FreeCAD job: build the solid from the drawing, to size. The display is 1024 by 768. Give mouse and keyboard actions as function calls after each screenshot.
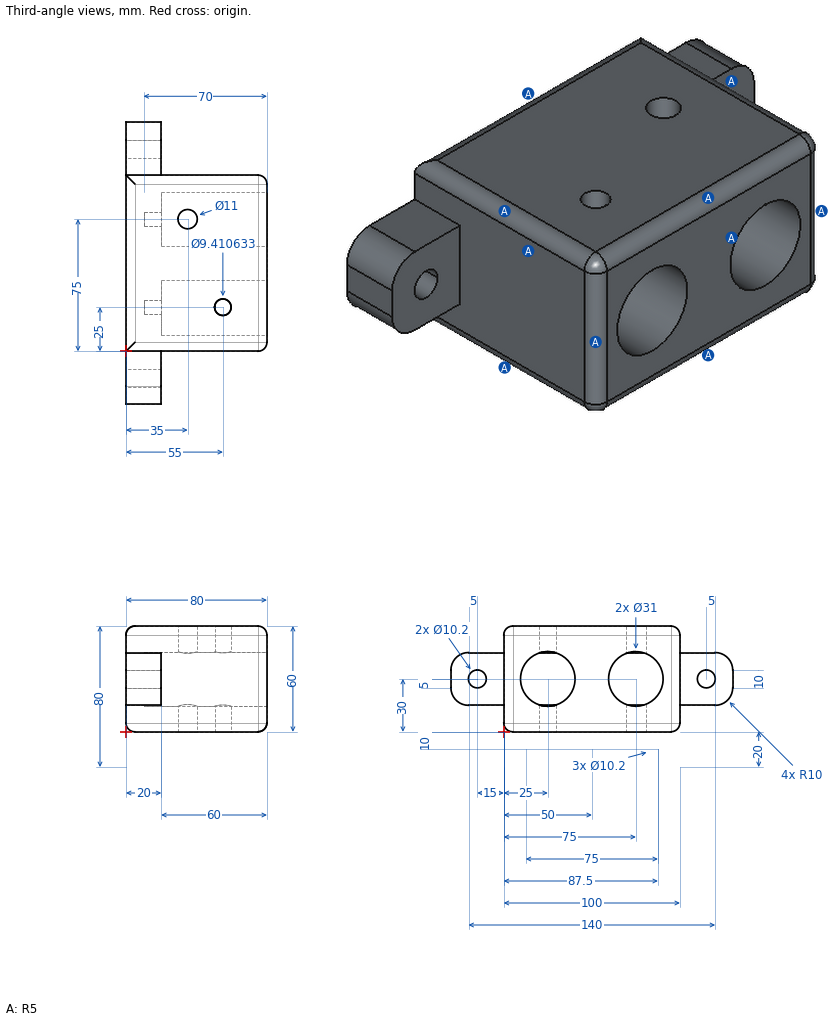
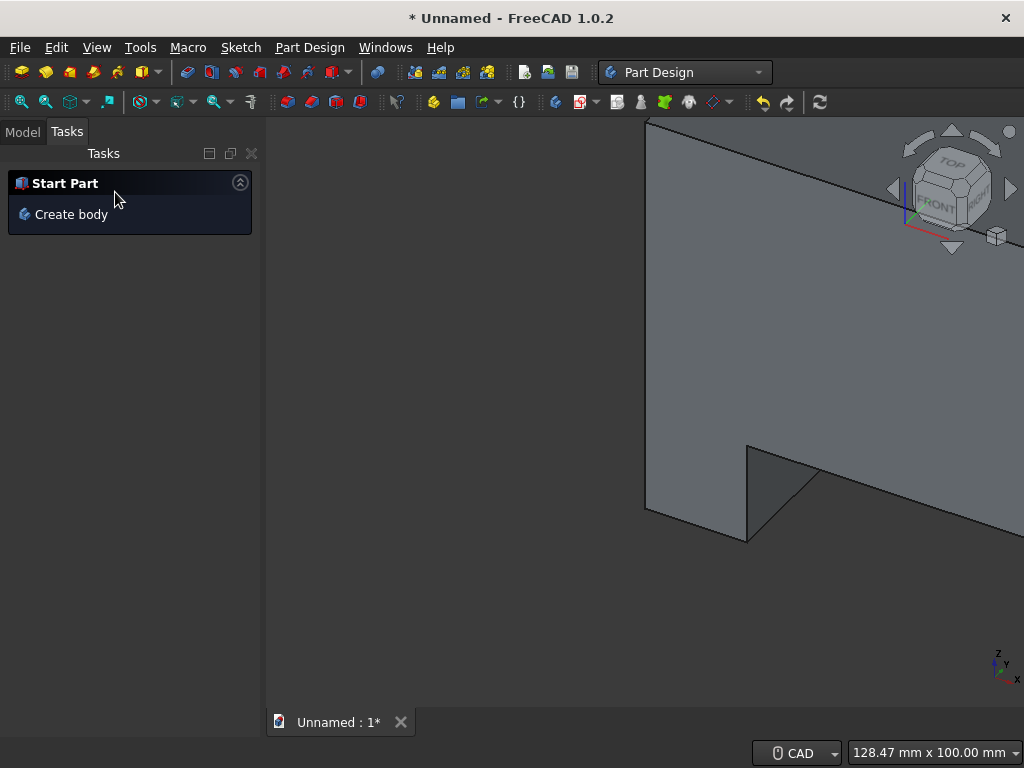
key(v)
key(f)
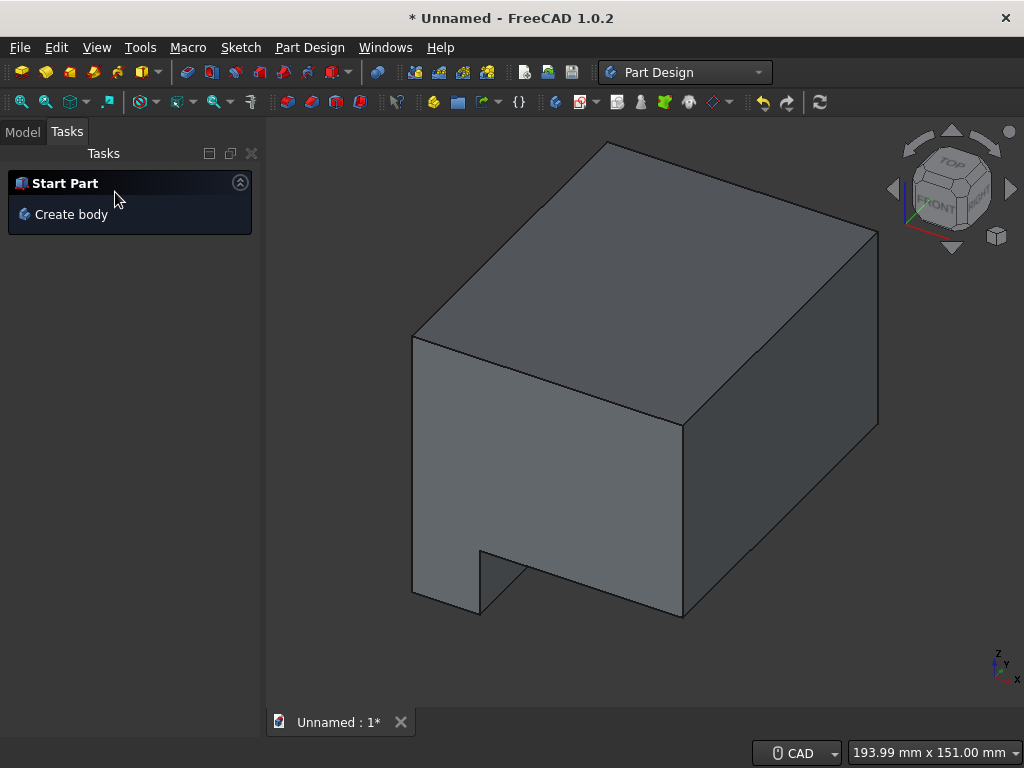
click(808, 396)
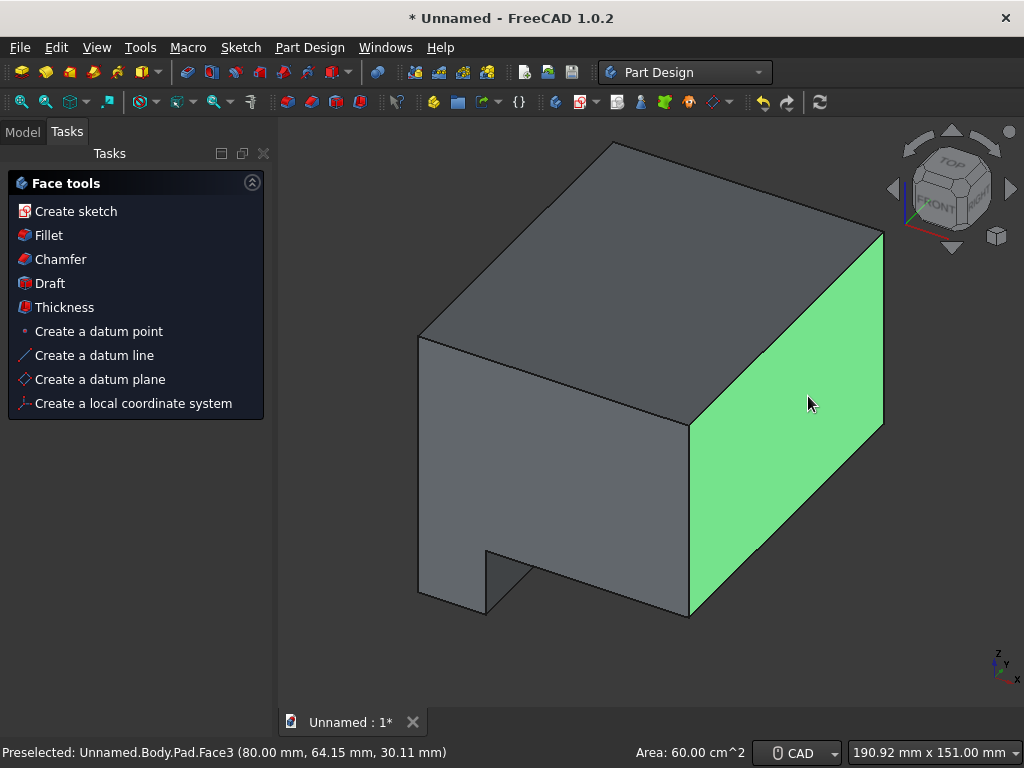
click(580, 102)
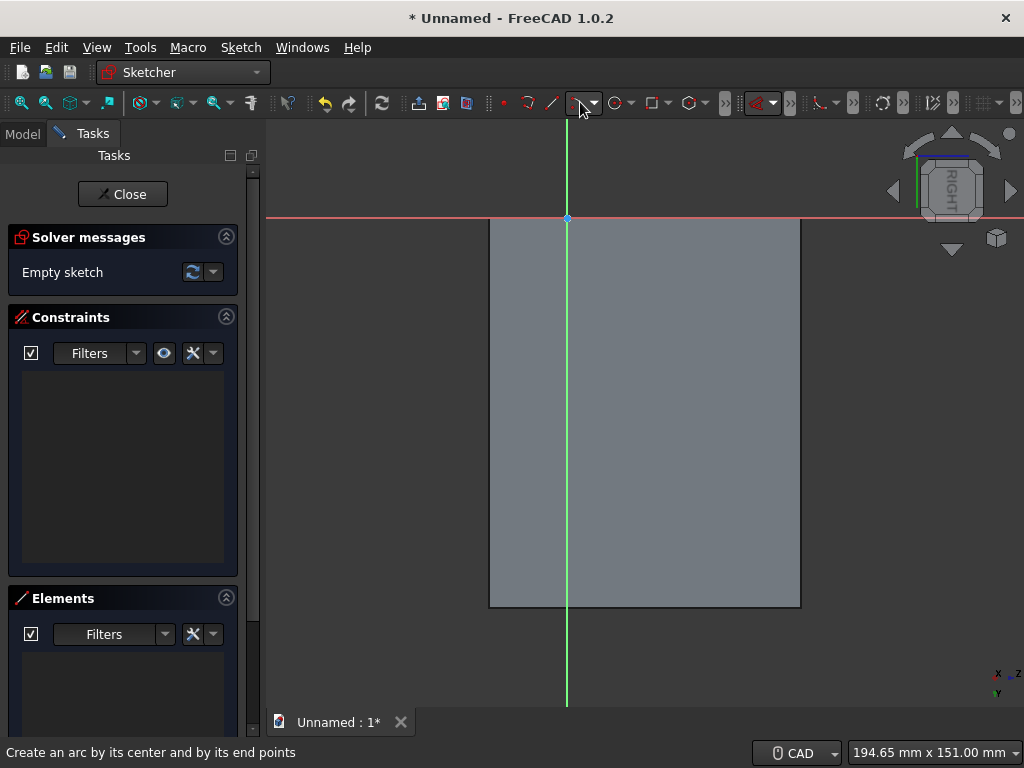
key(g)
key(c)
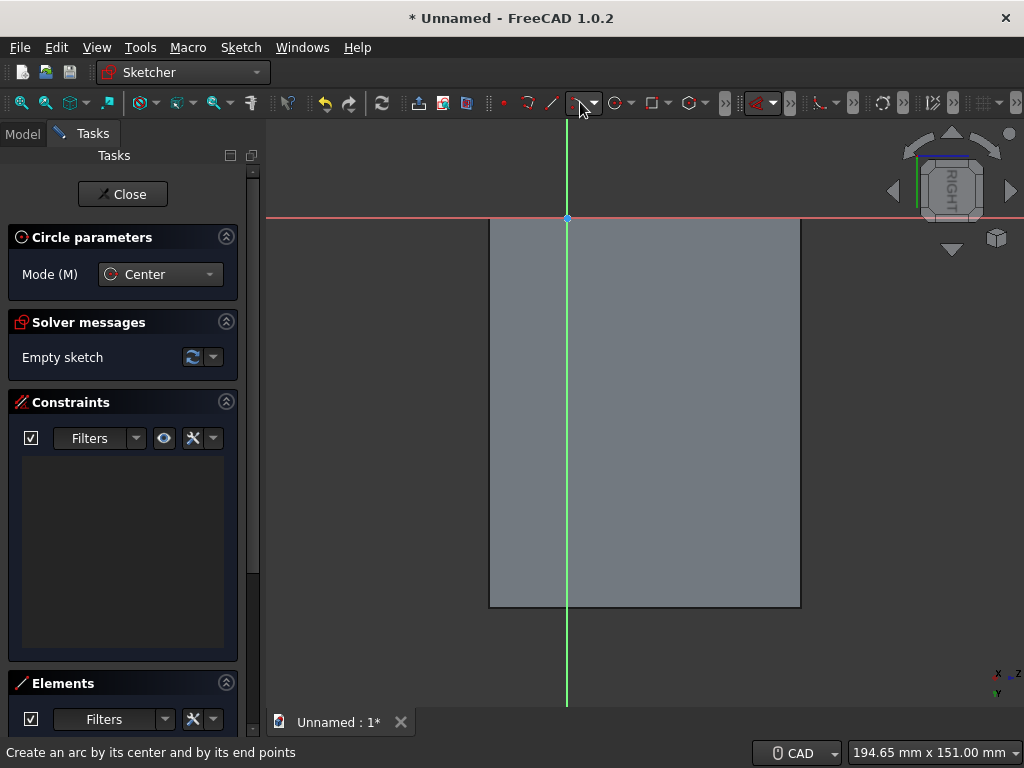
click(684, 510)
move(727, 468)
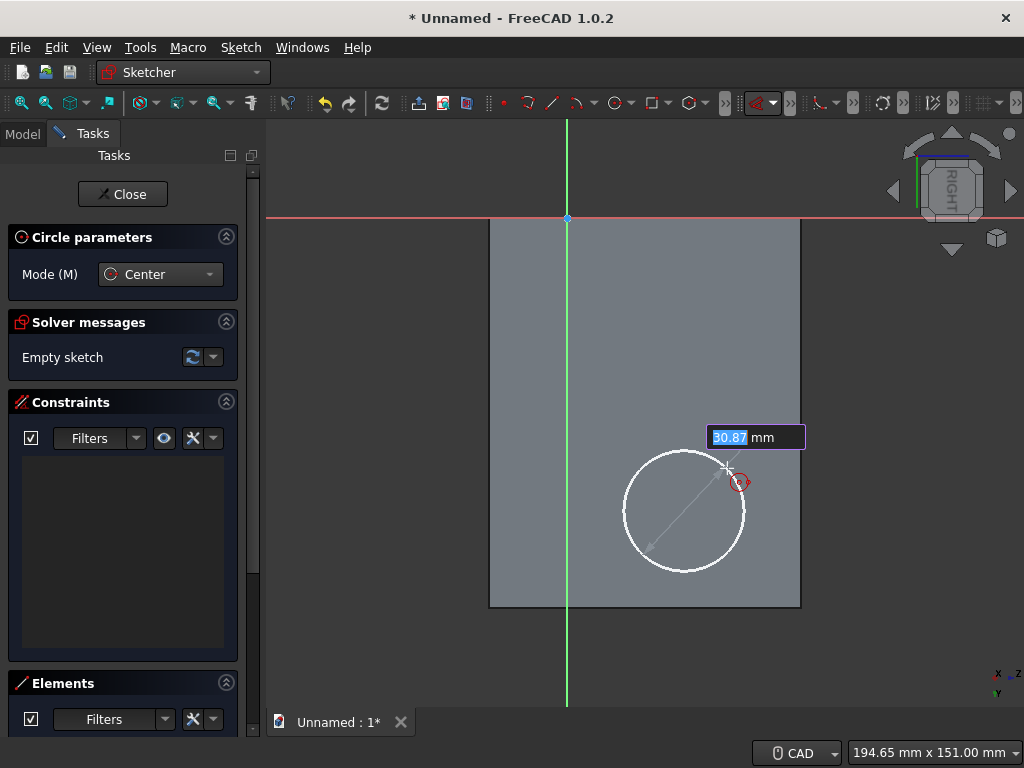
text(31)
key(Return)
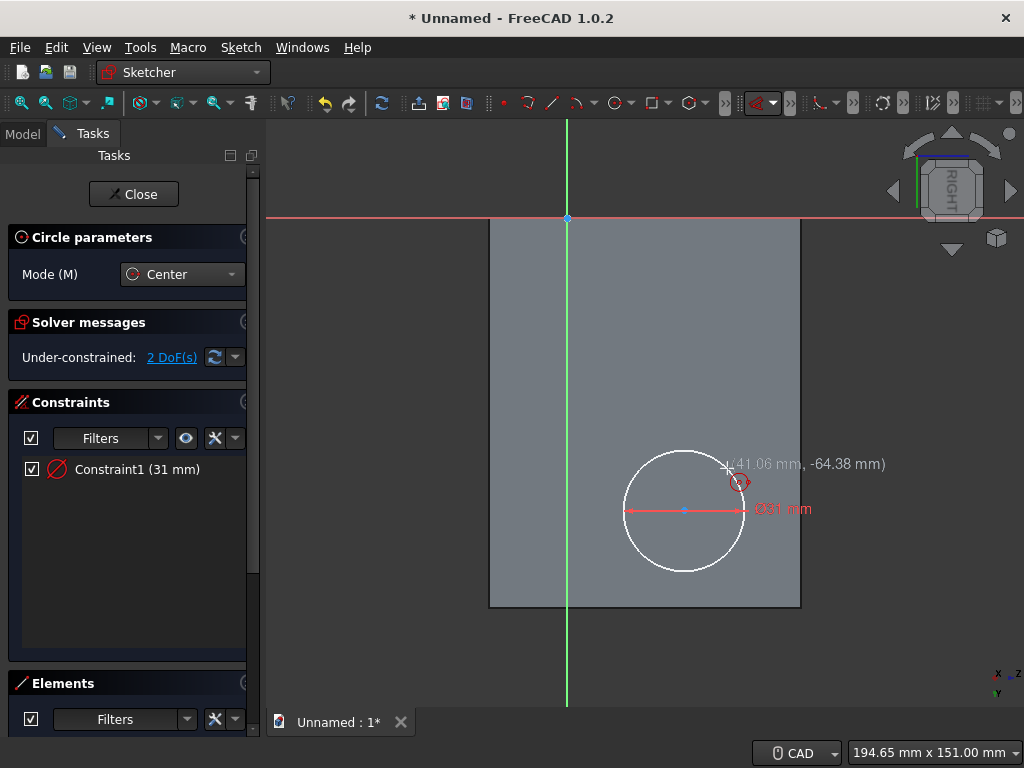
click(684, 316)
move(727, 273)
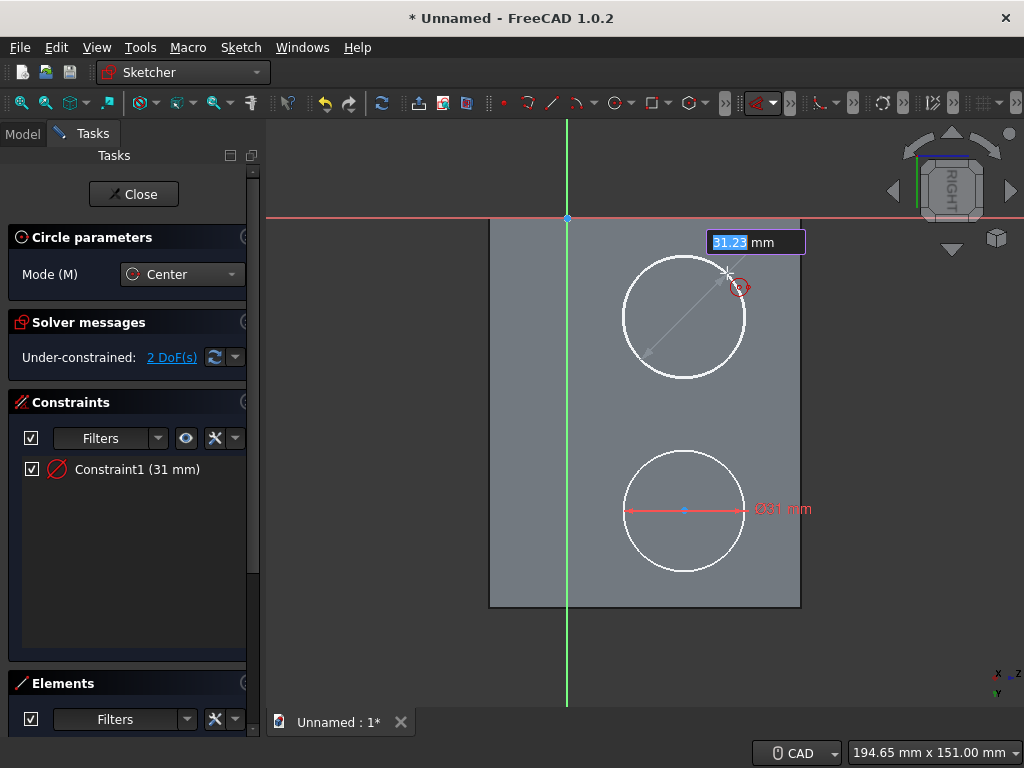
text(31)
key(Return)
key(Escape)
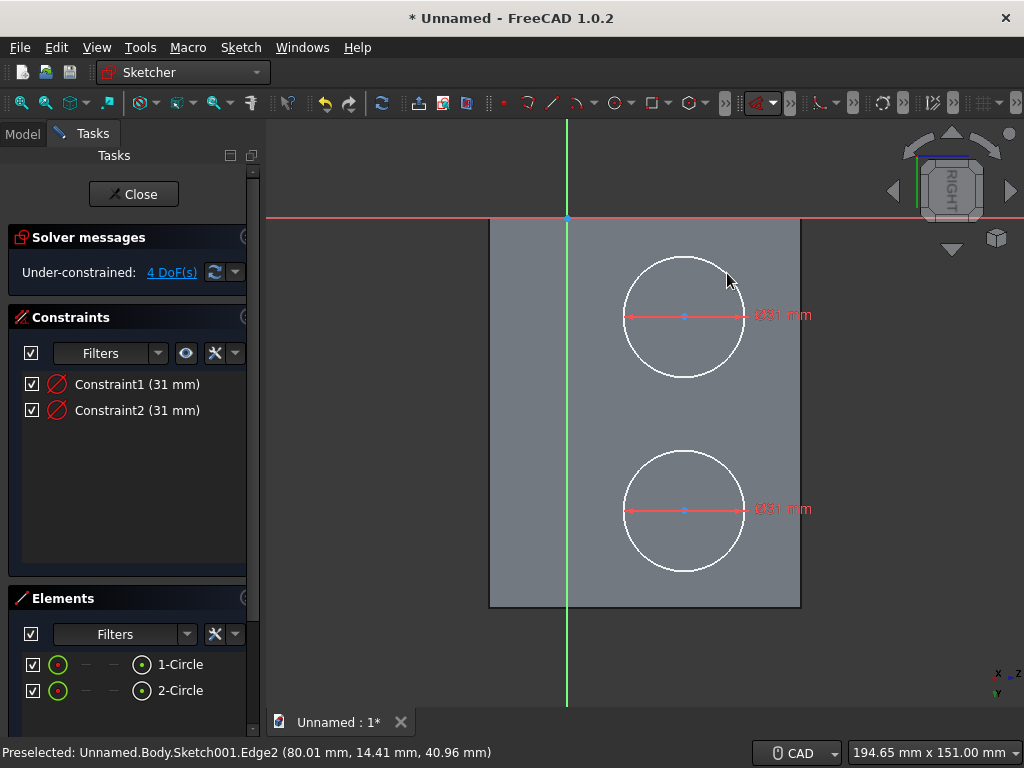
click(684, 511)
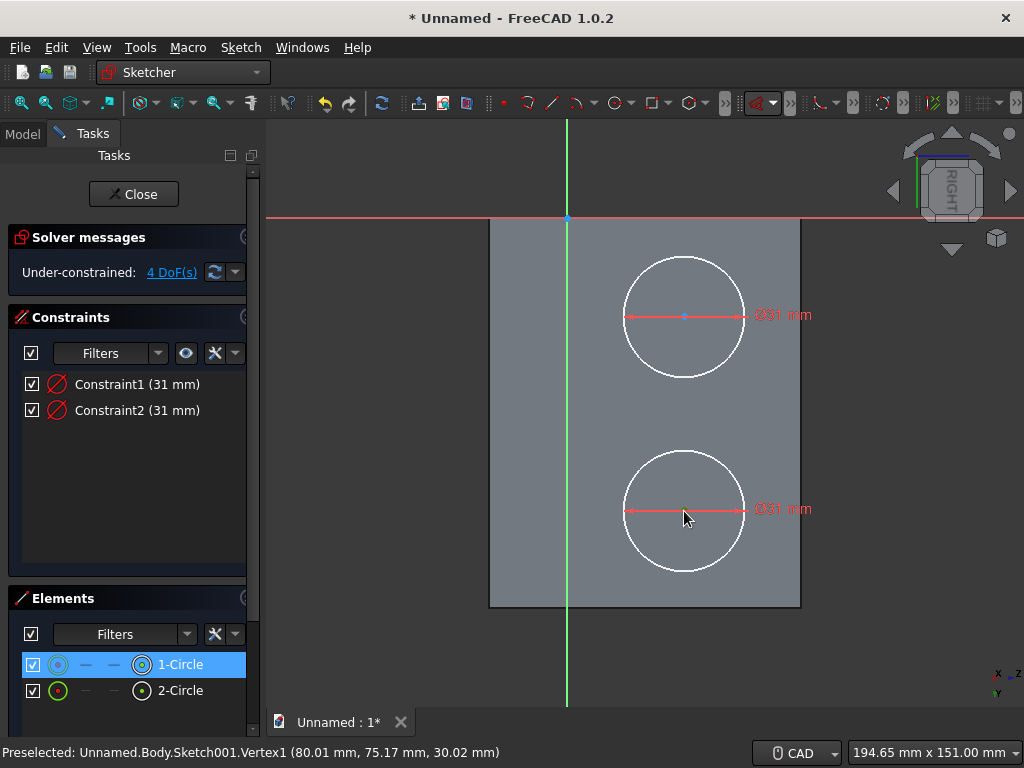
click(684, 317)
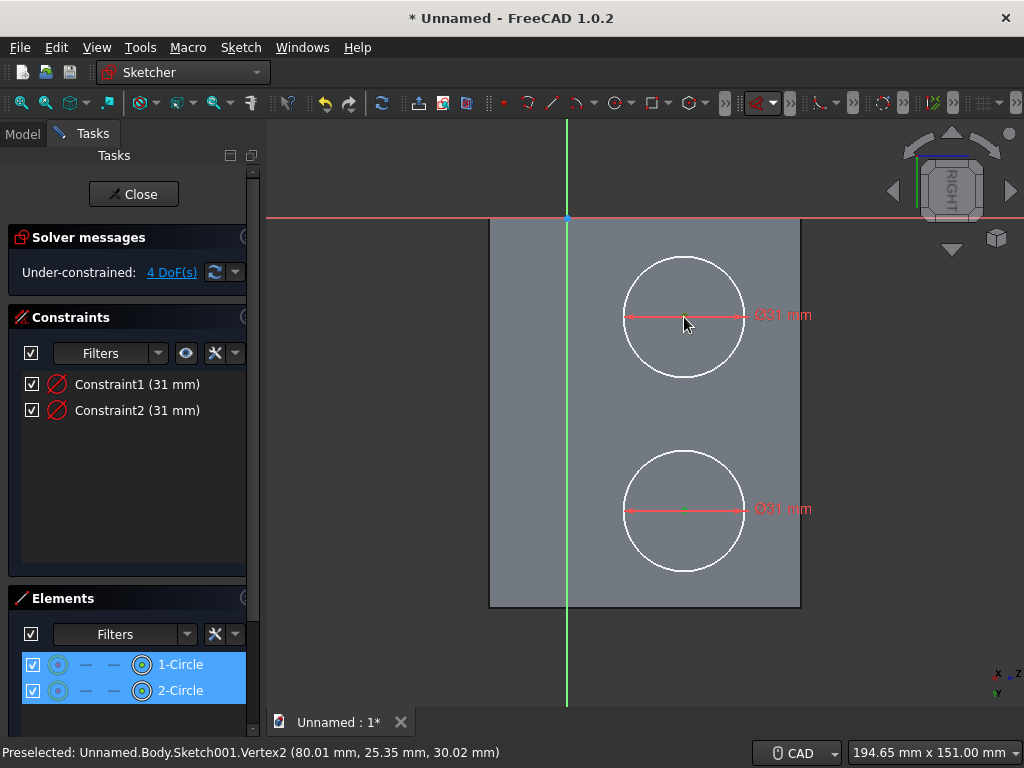
key(v)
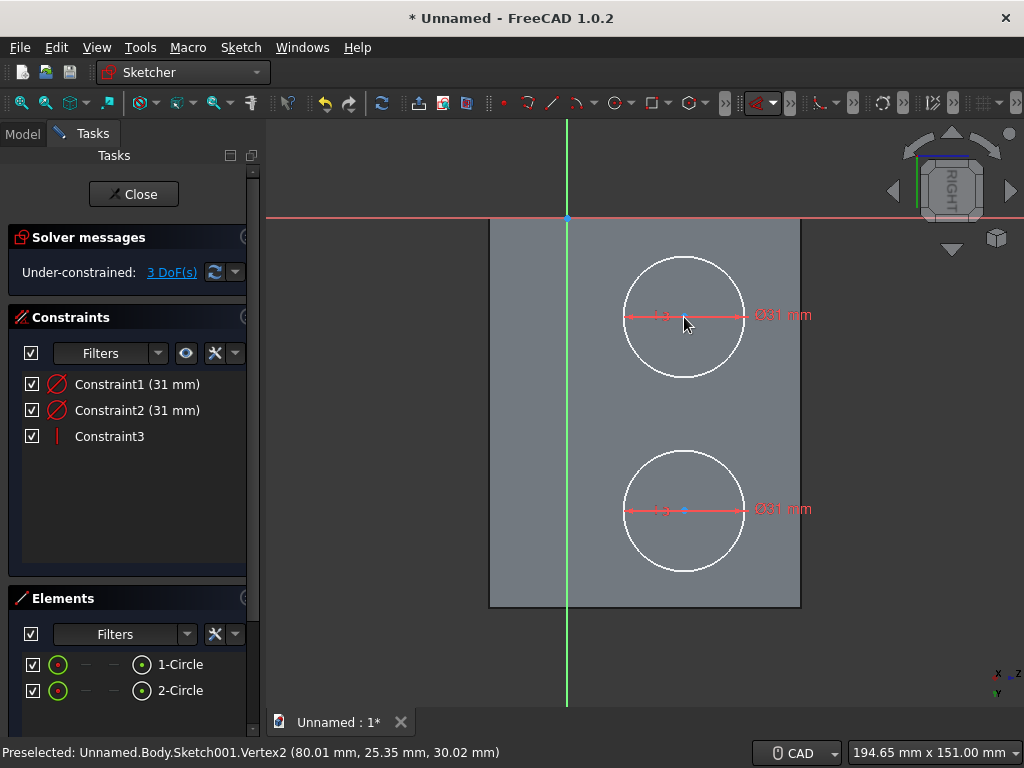
click(684, 511)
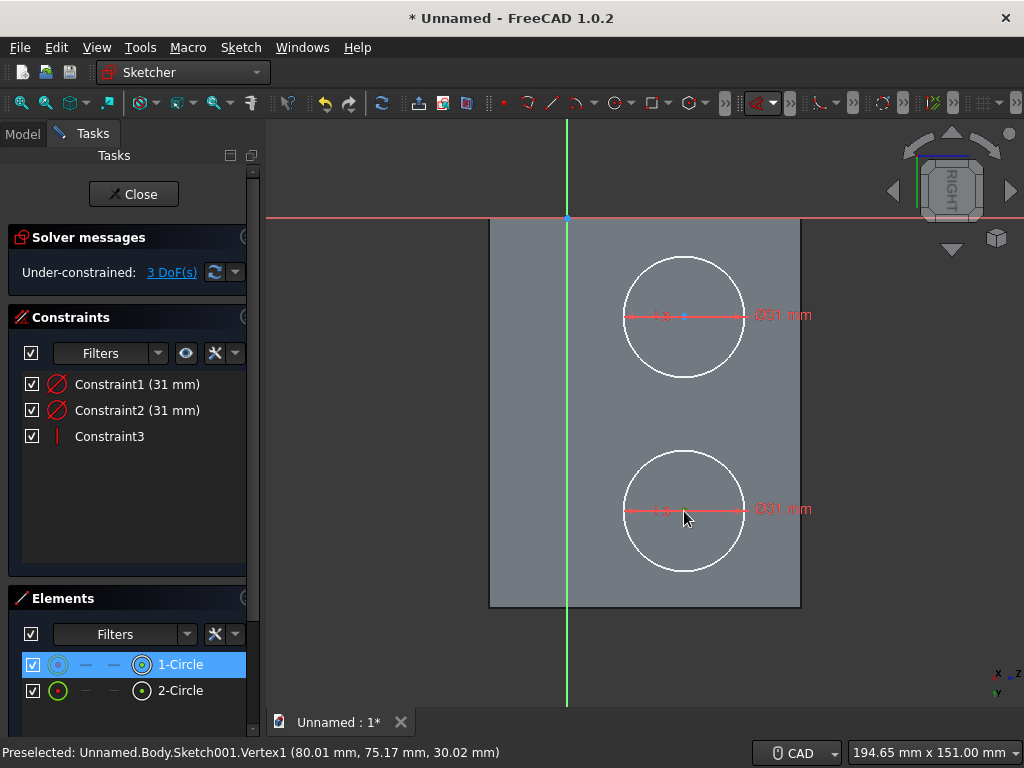
key(l)